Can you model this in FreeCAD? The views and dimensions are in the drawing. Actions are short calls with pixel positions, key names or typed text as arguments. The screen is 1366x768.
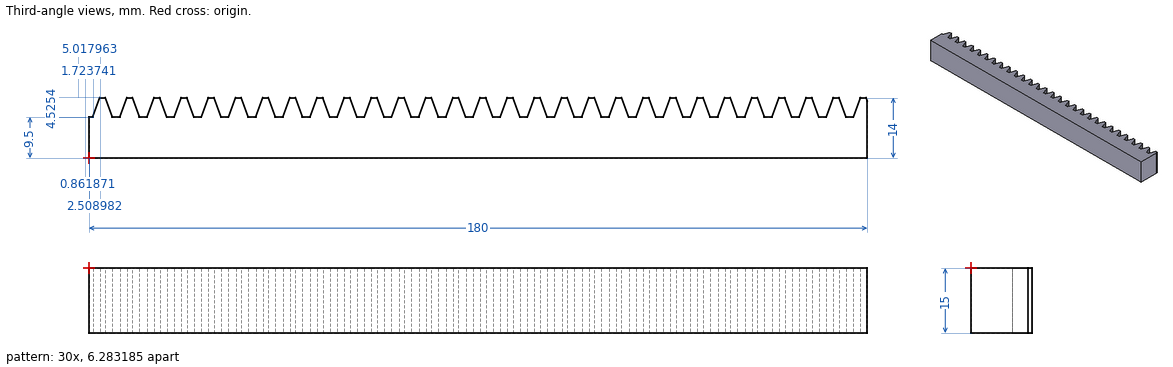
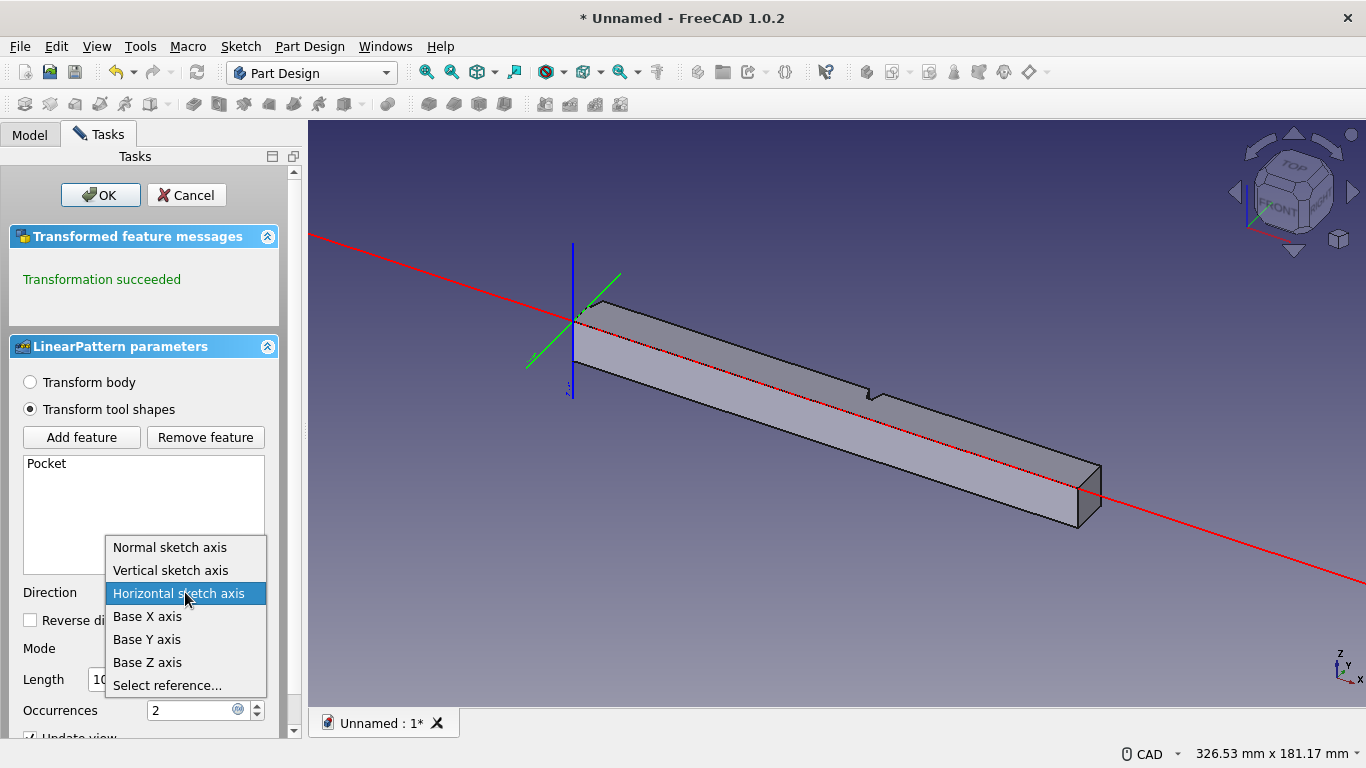
click(184, 616)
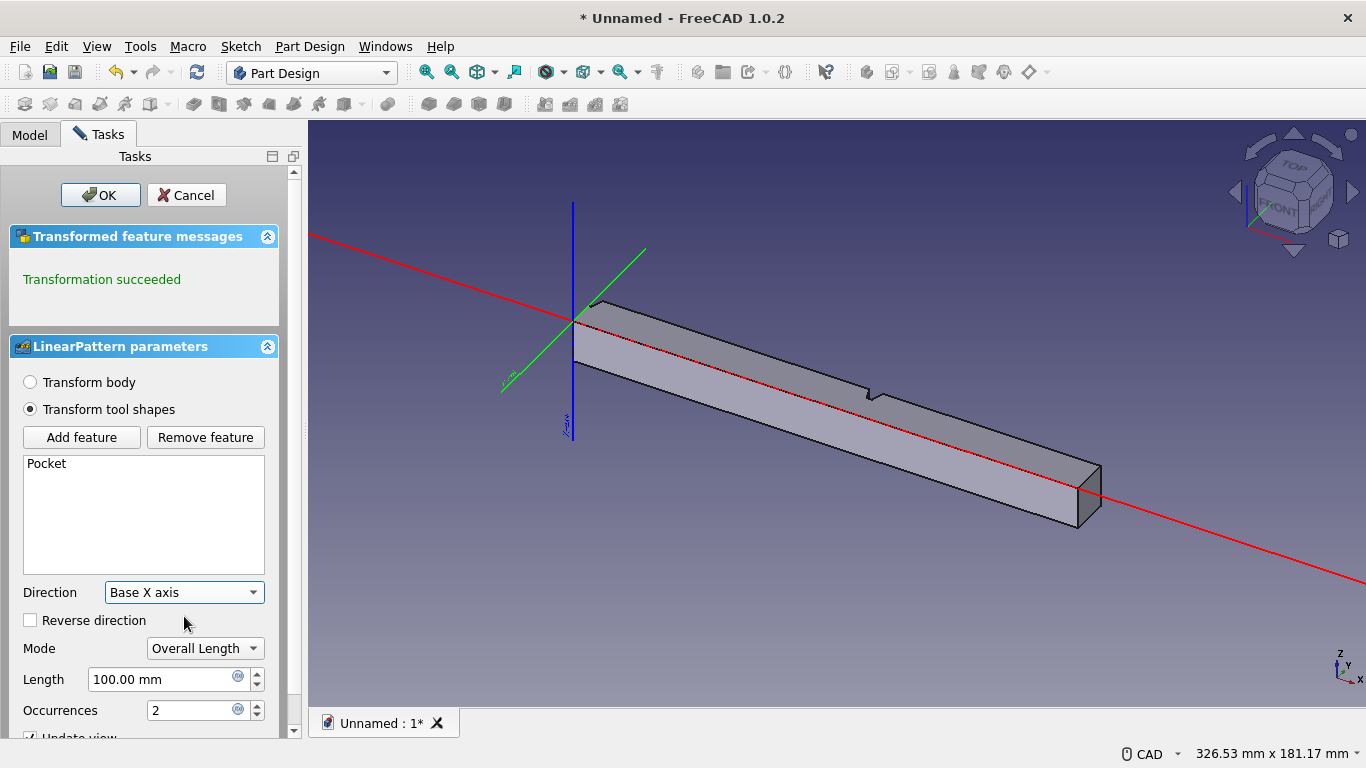
click(206, 648)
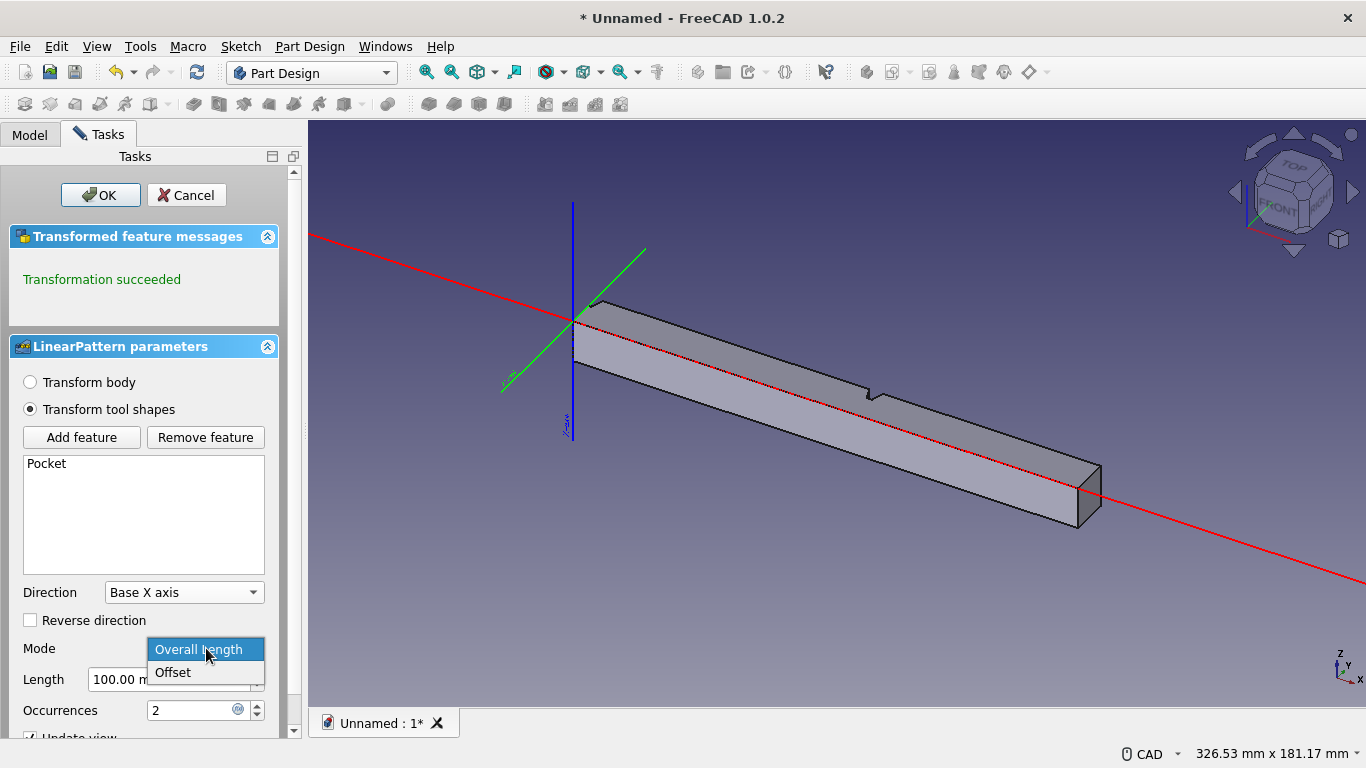
click(204, 672)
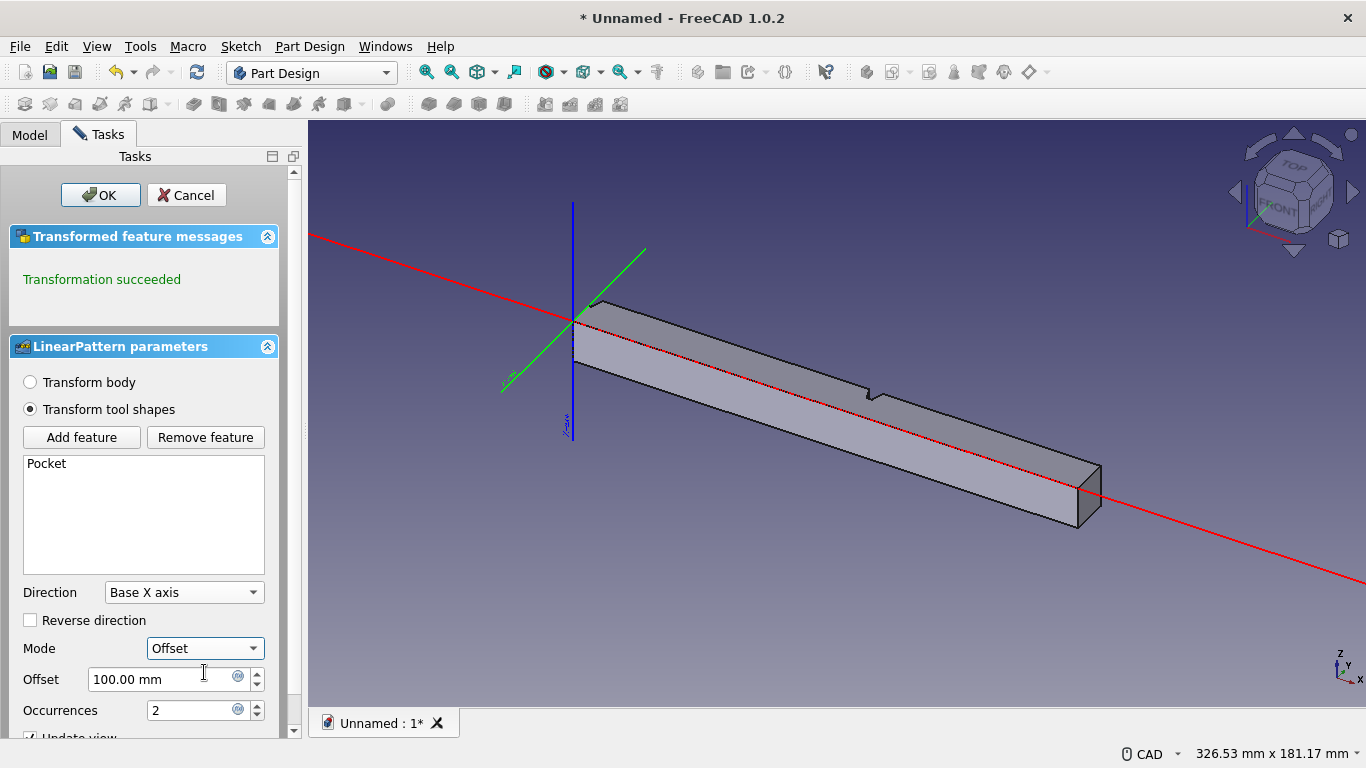
triple_click(170, 680)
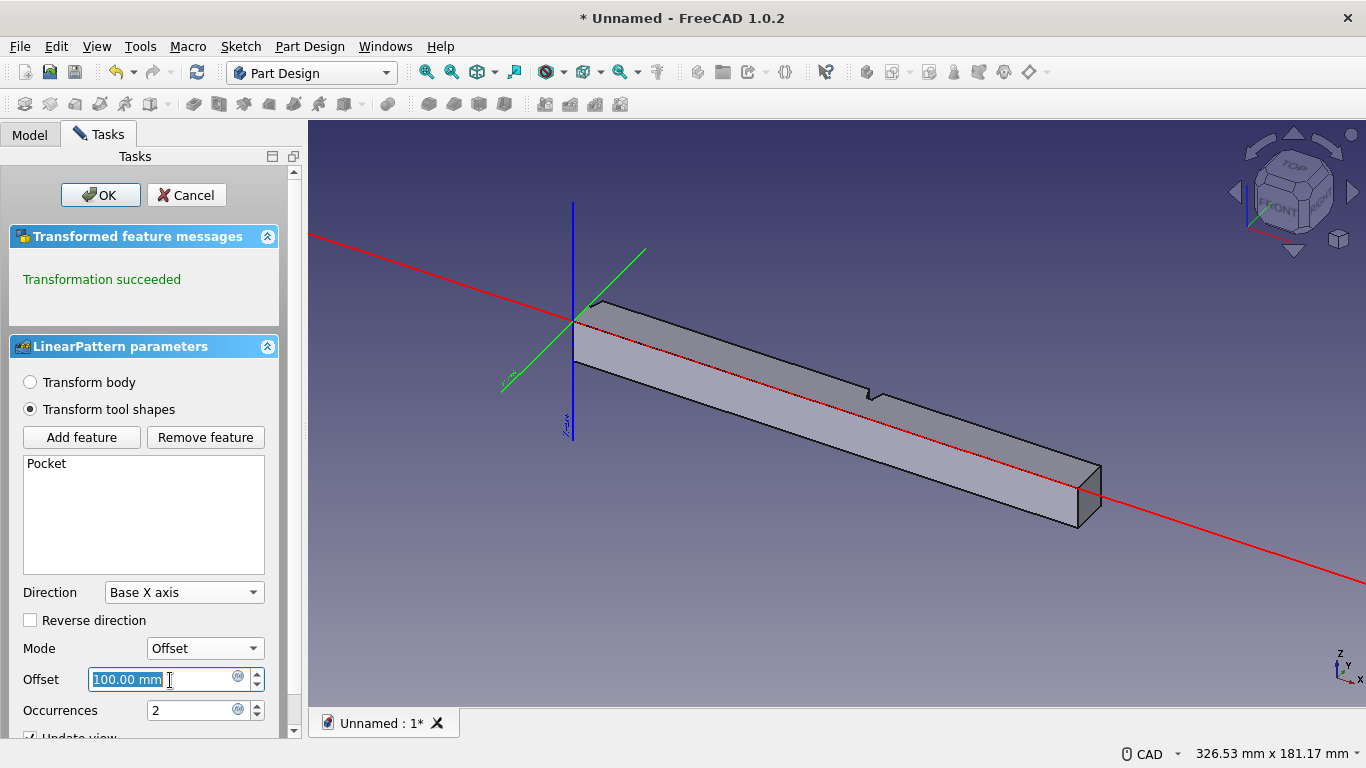
text(6.283185)
key(Tab)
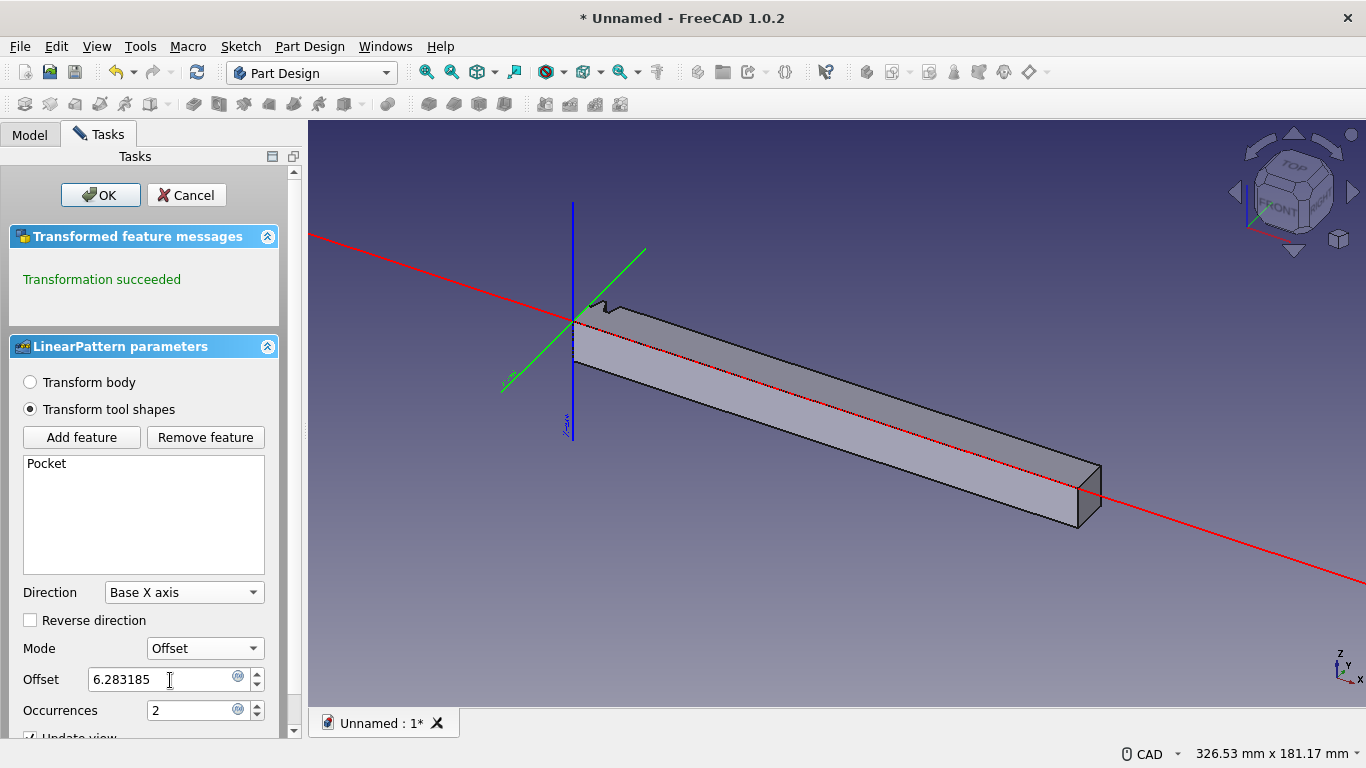
triple_click(199, 710)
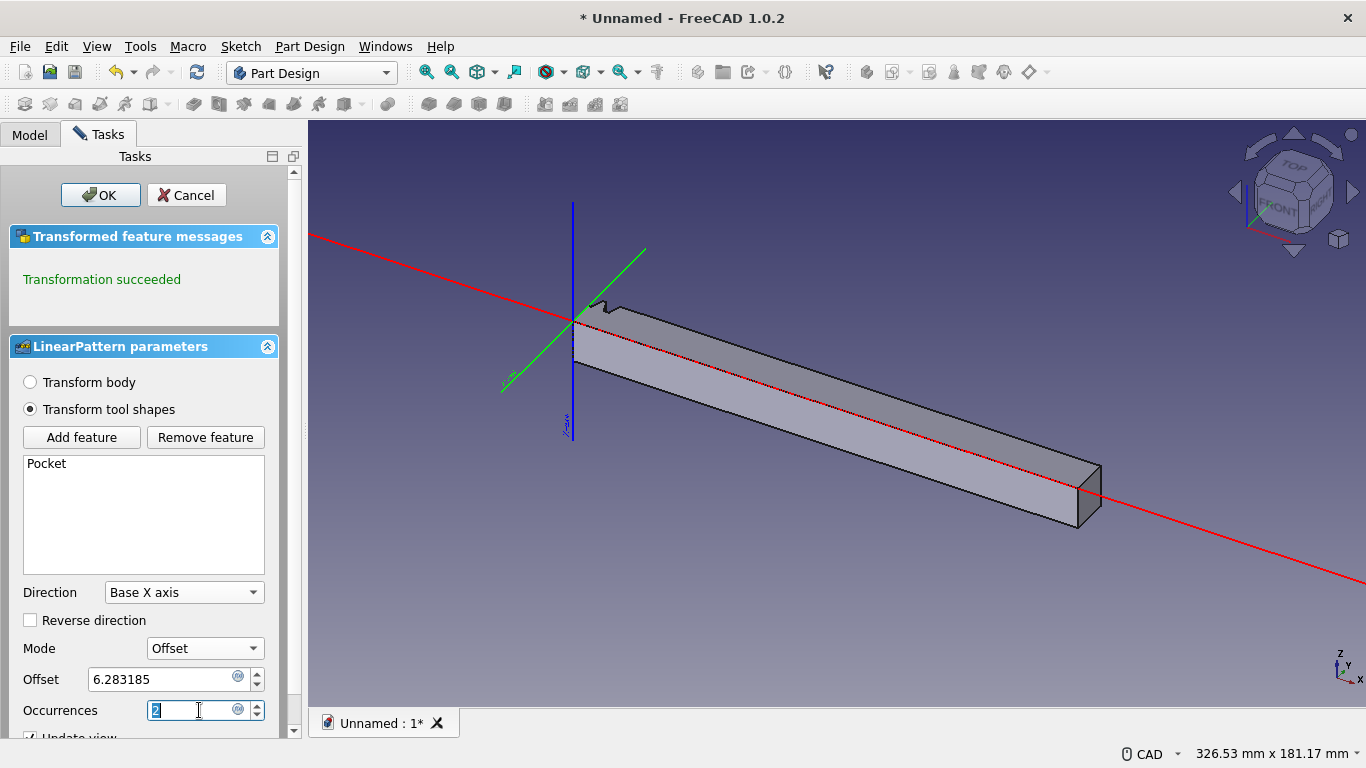
text(30)
key(Tab)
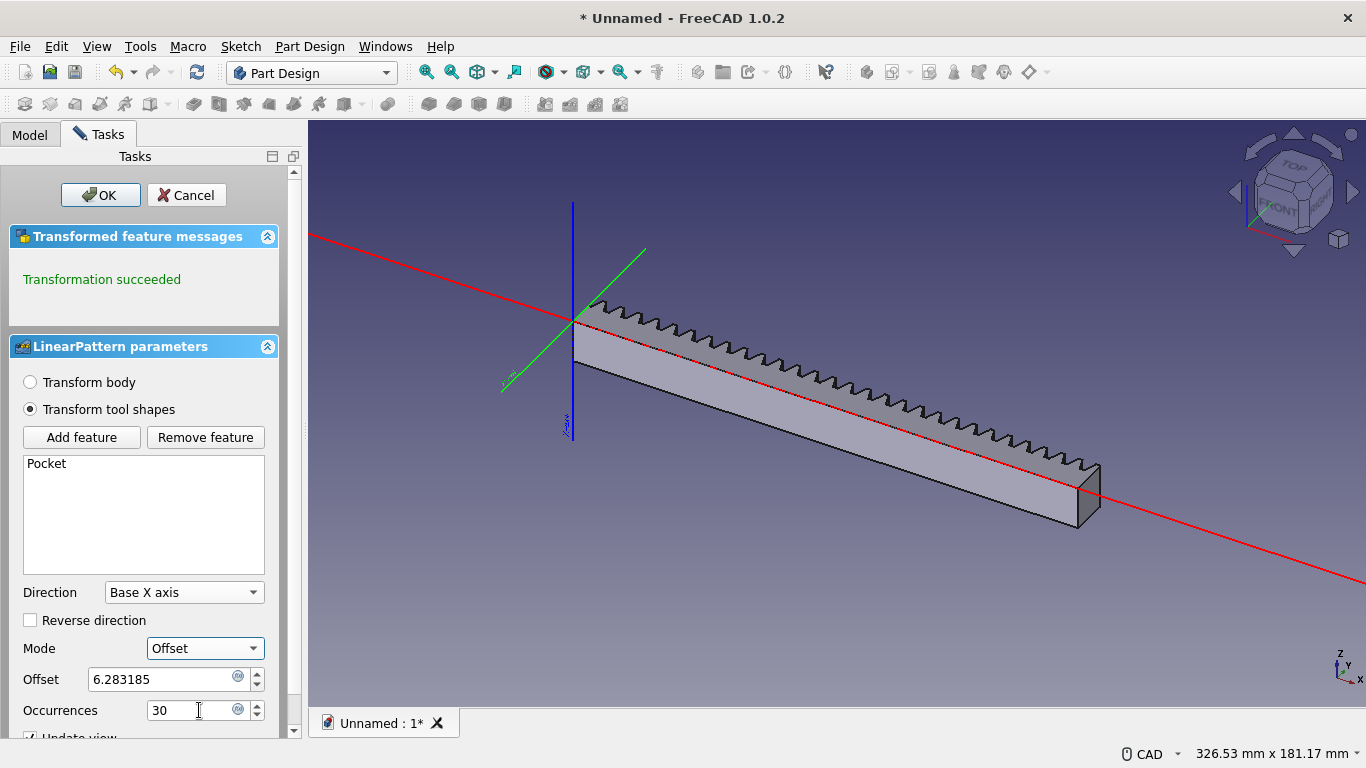
click(101, 195)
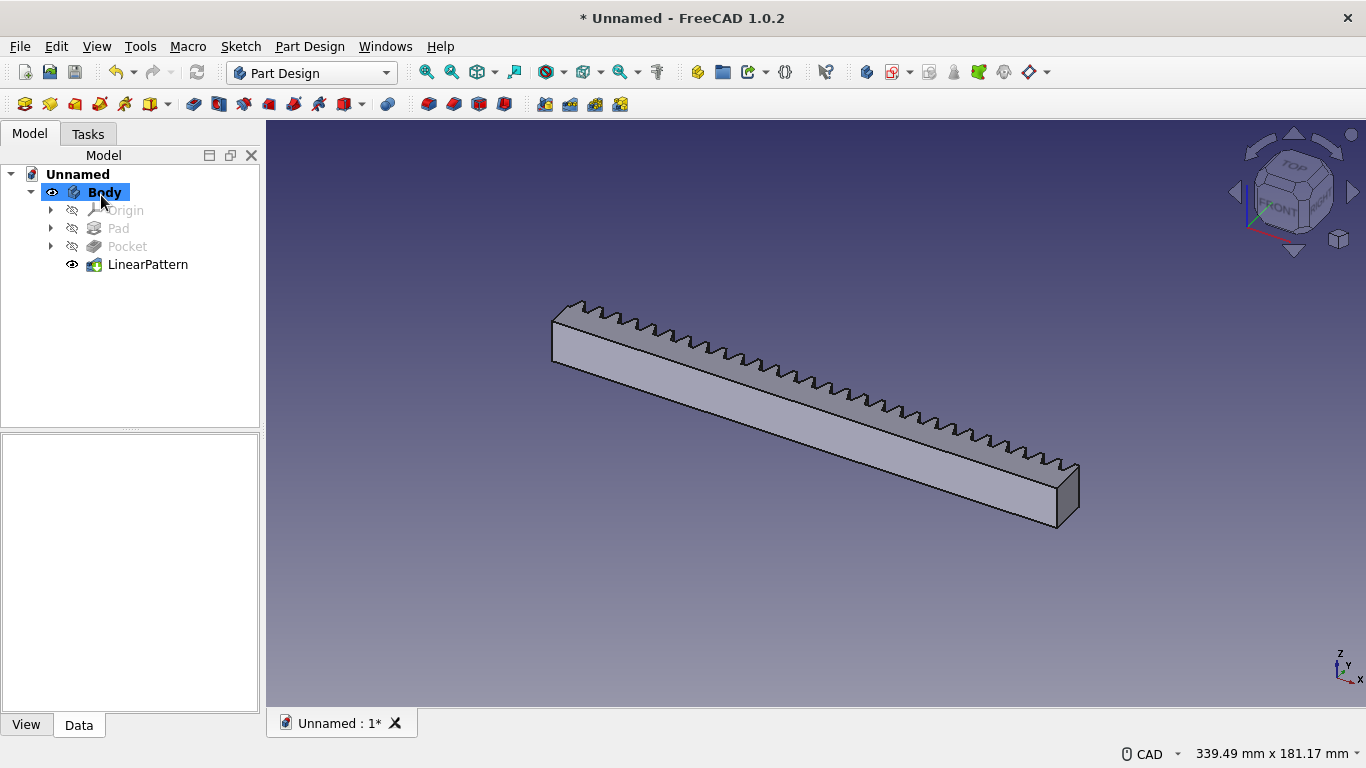
key(0)